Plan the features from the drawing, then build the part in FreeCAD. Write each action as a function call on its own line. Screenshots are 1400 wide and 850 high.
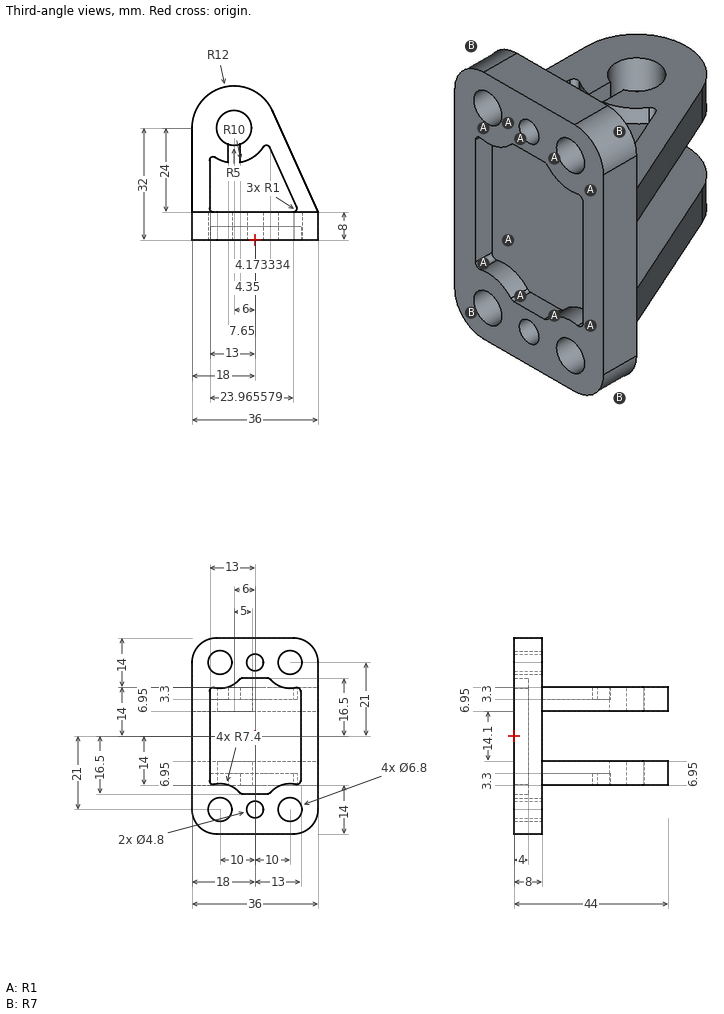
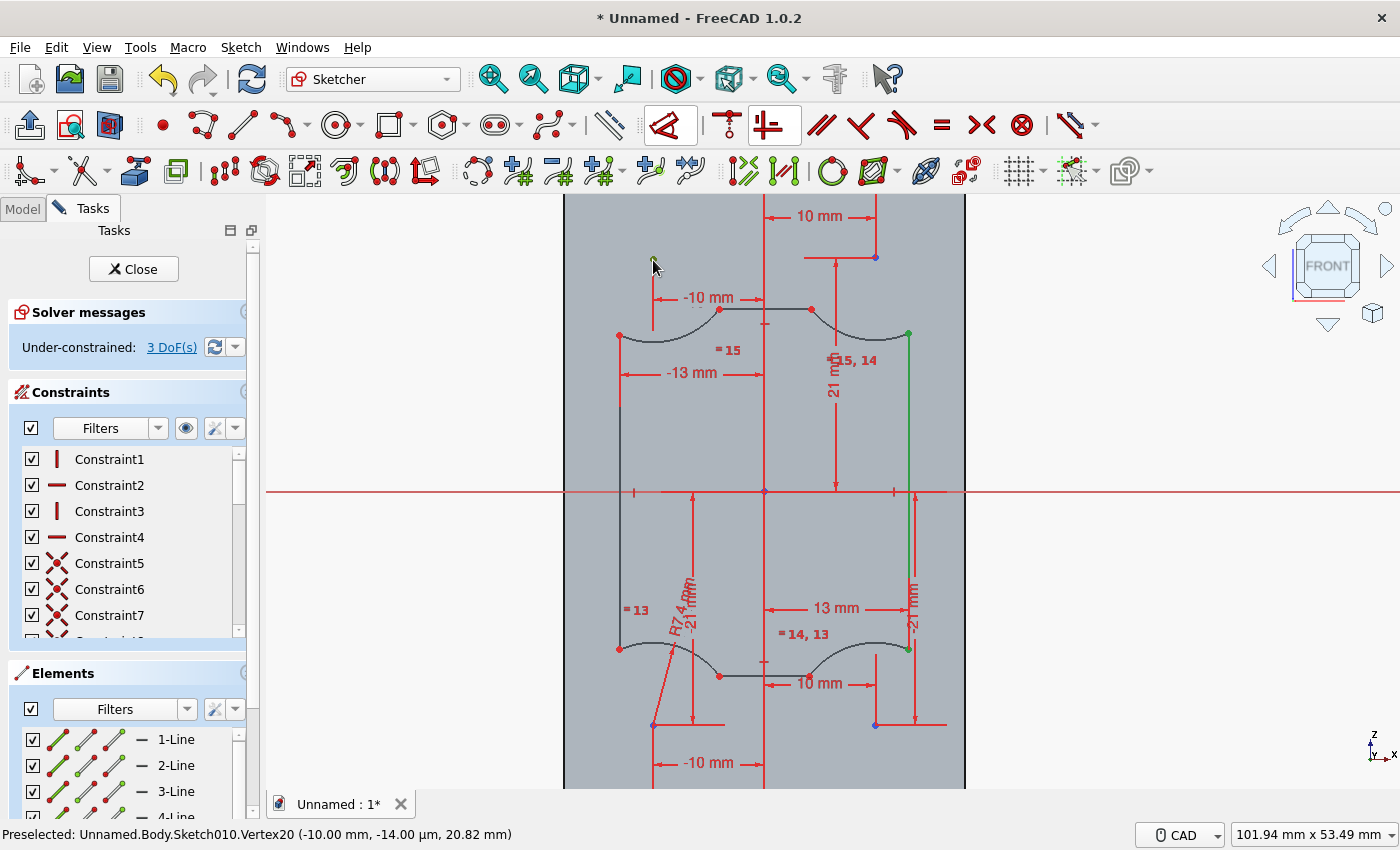
key(i)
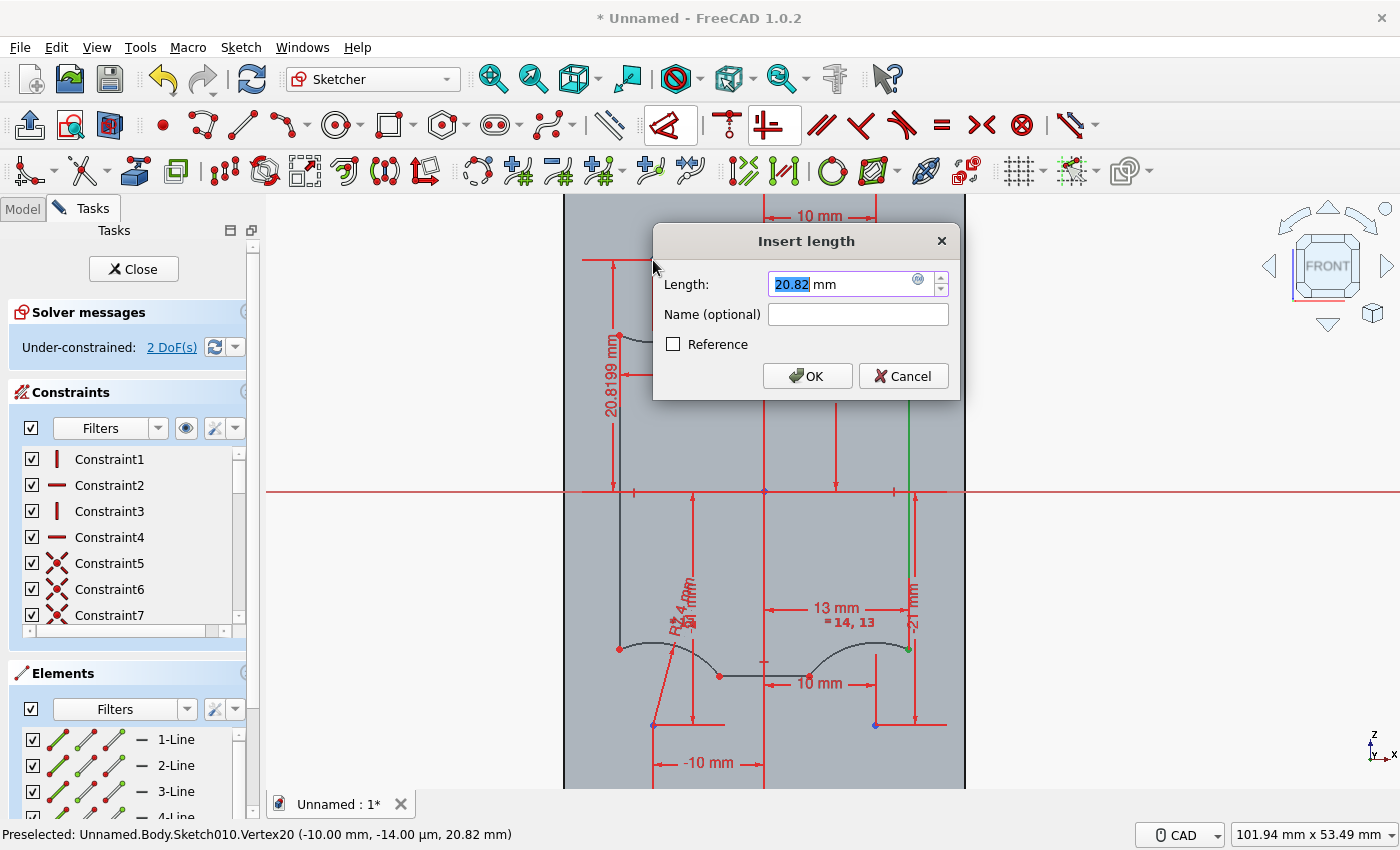
text(21)
key(Return)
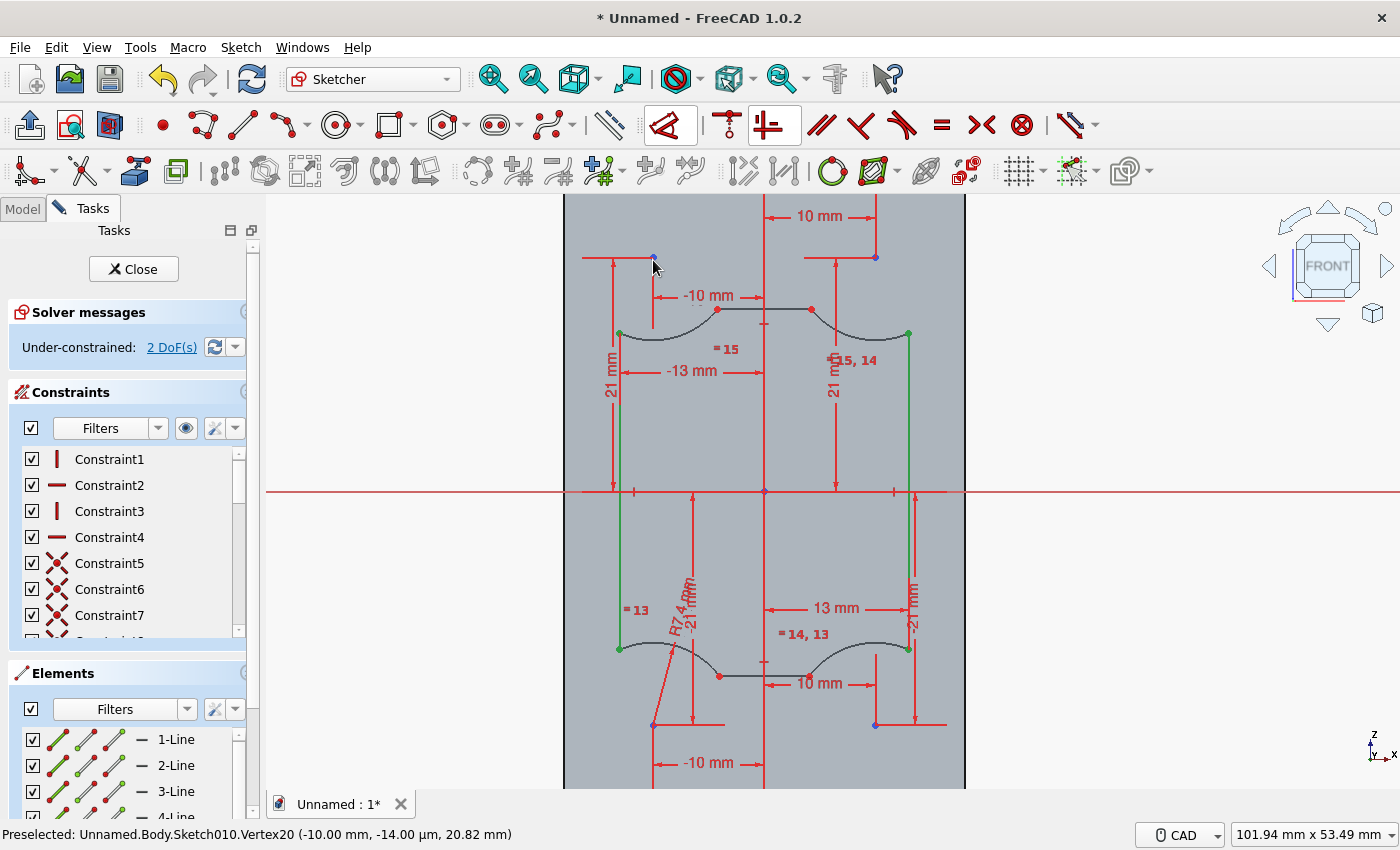
click(719, 676)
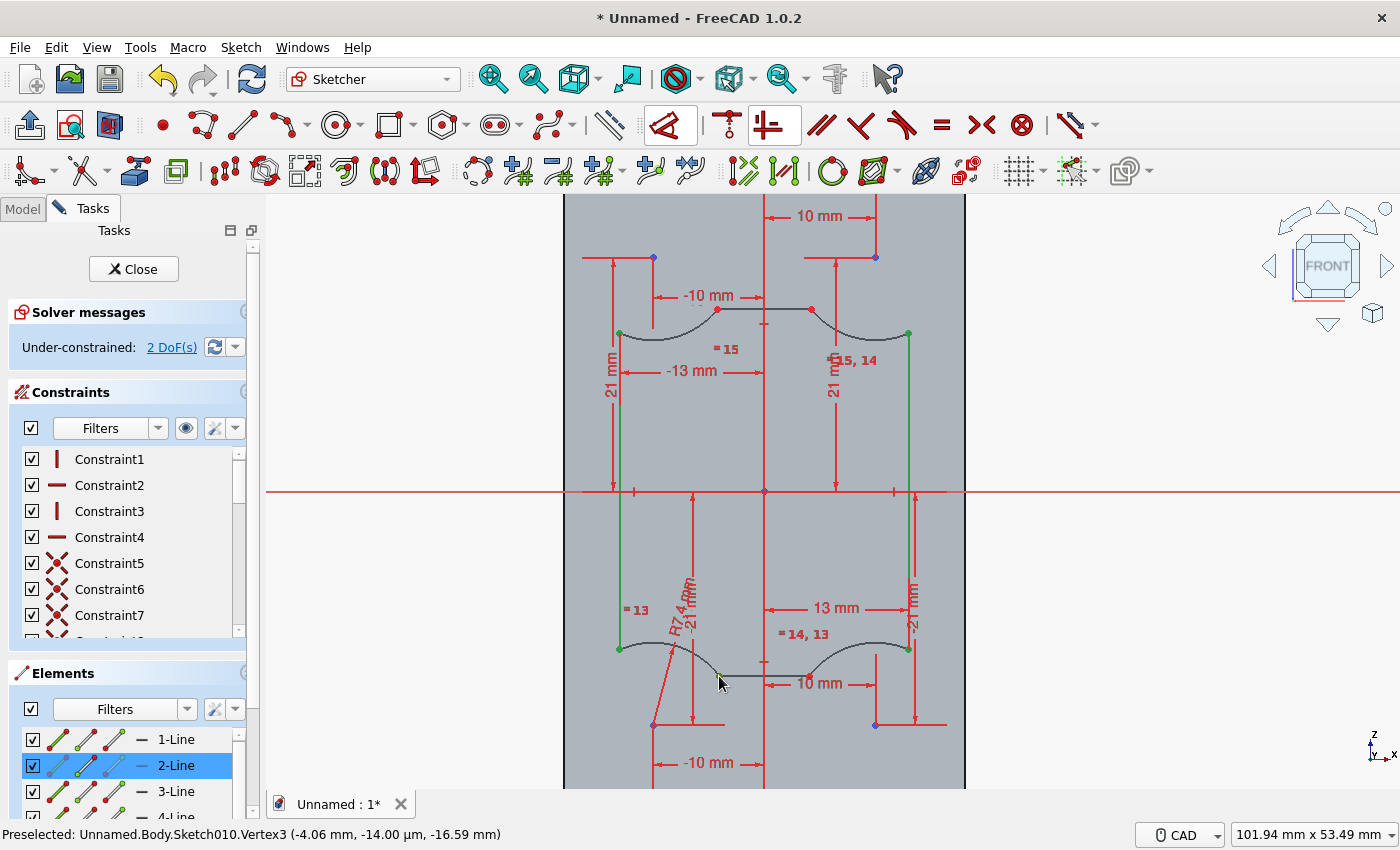
key(i)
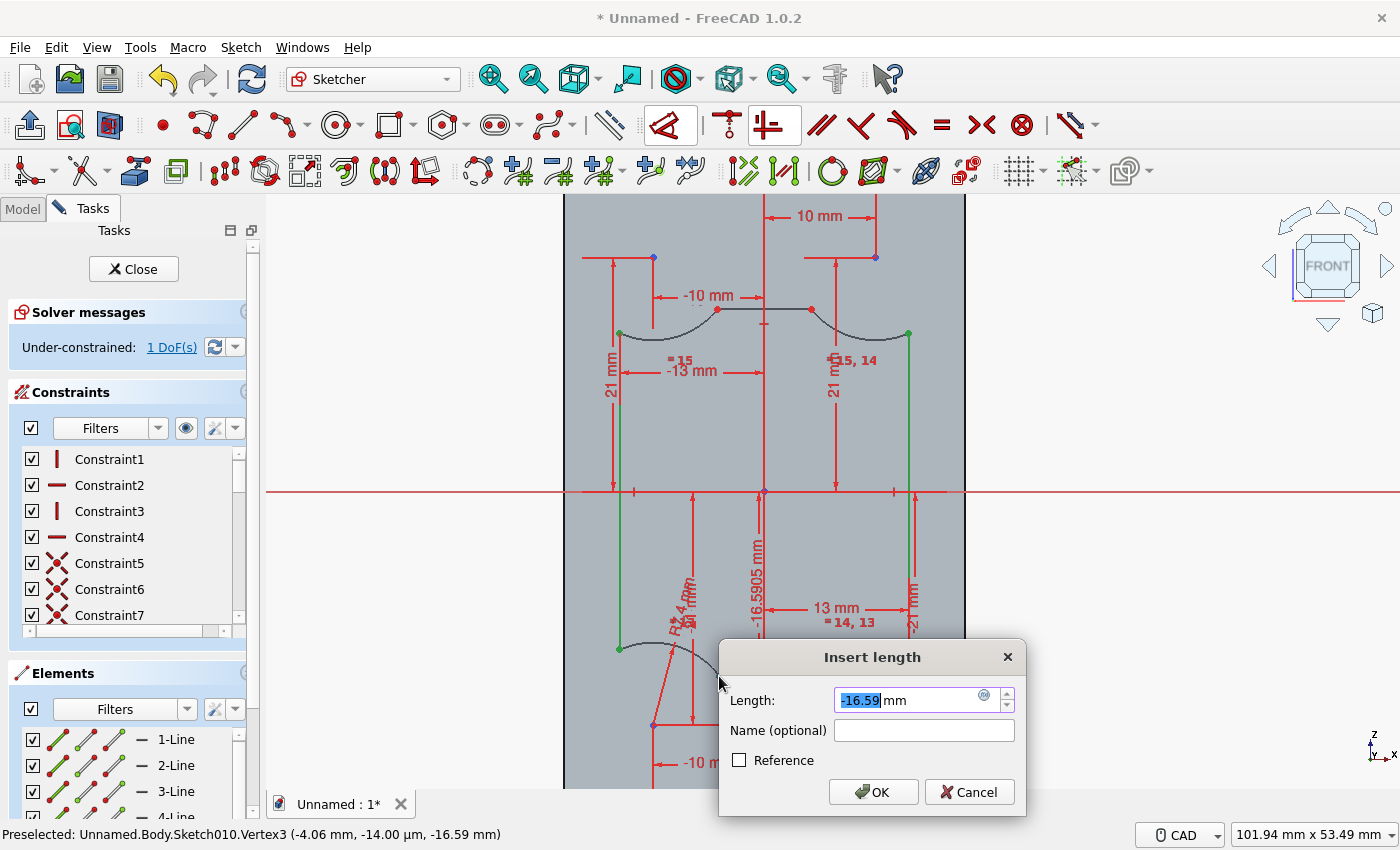
text(-16.5)
key(Return)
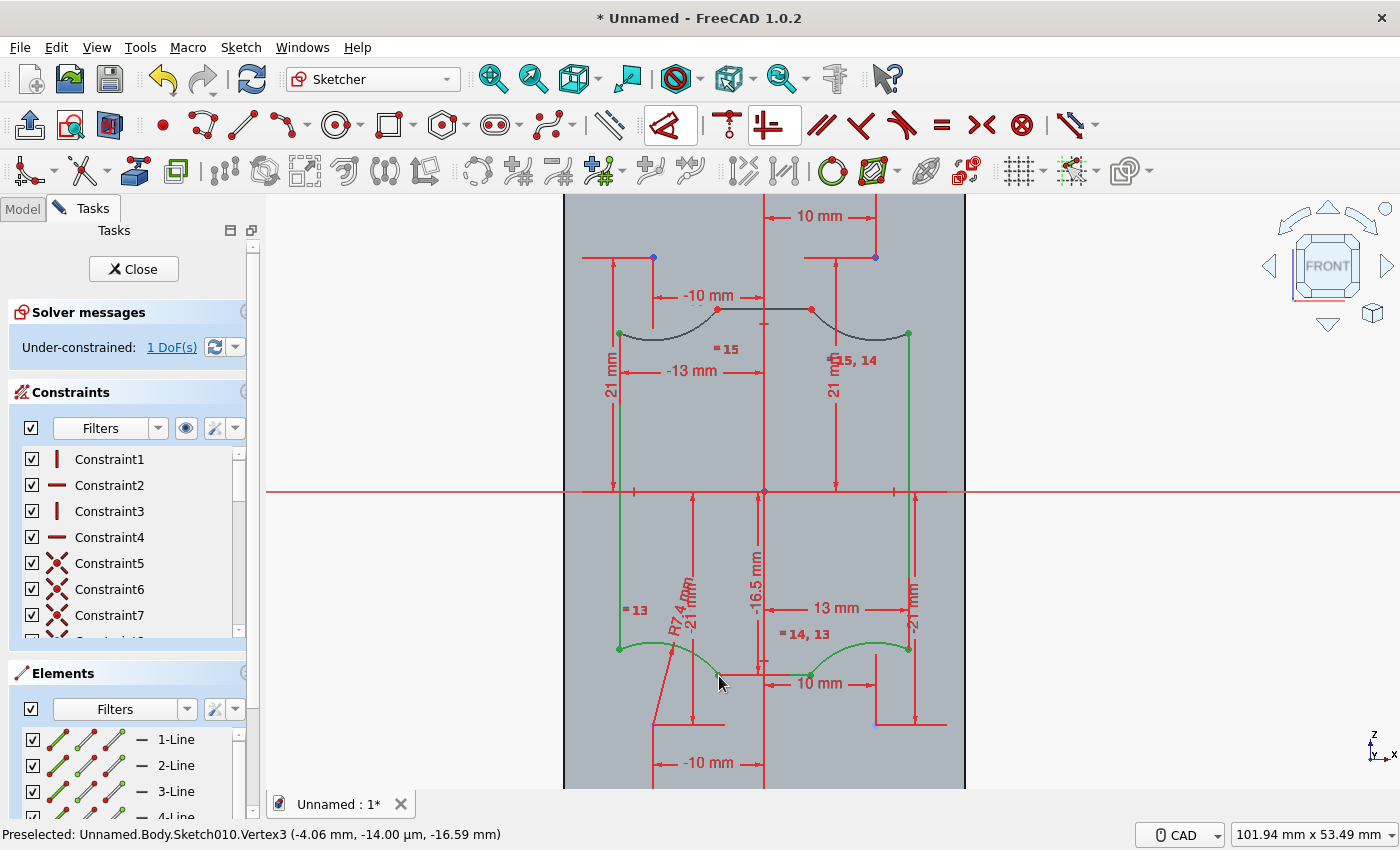
click(811, 309)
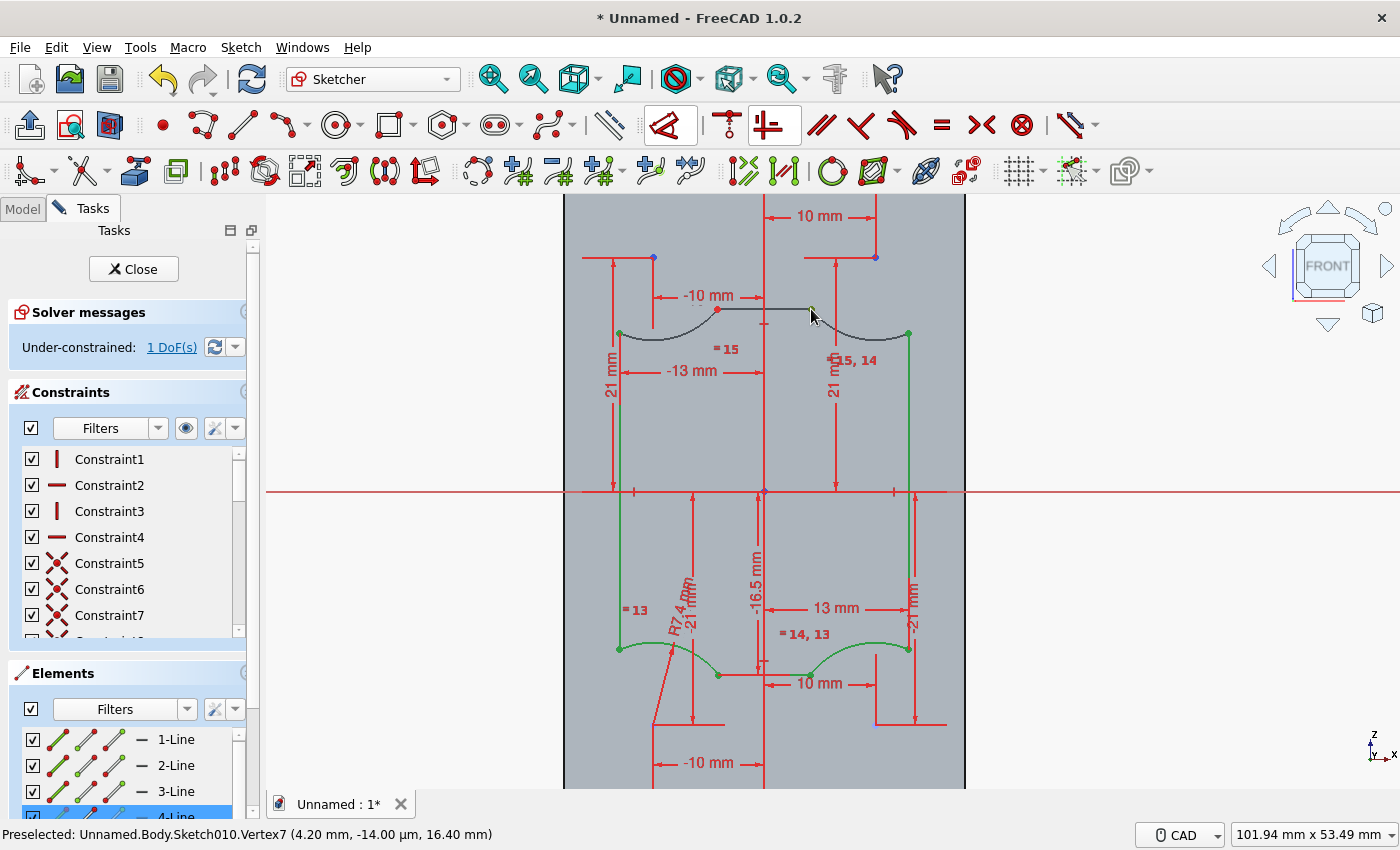
key(i)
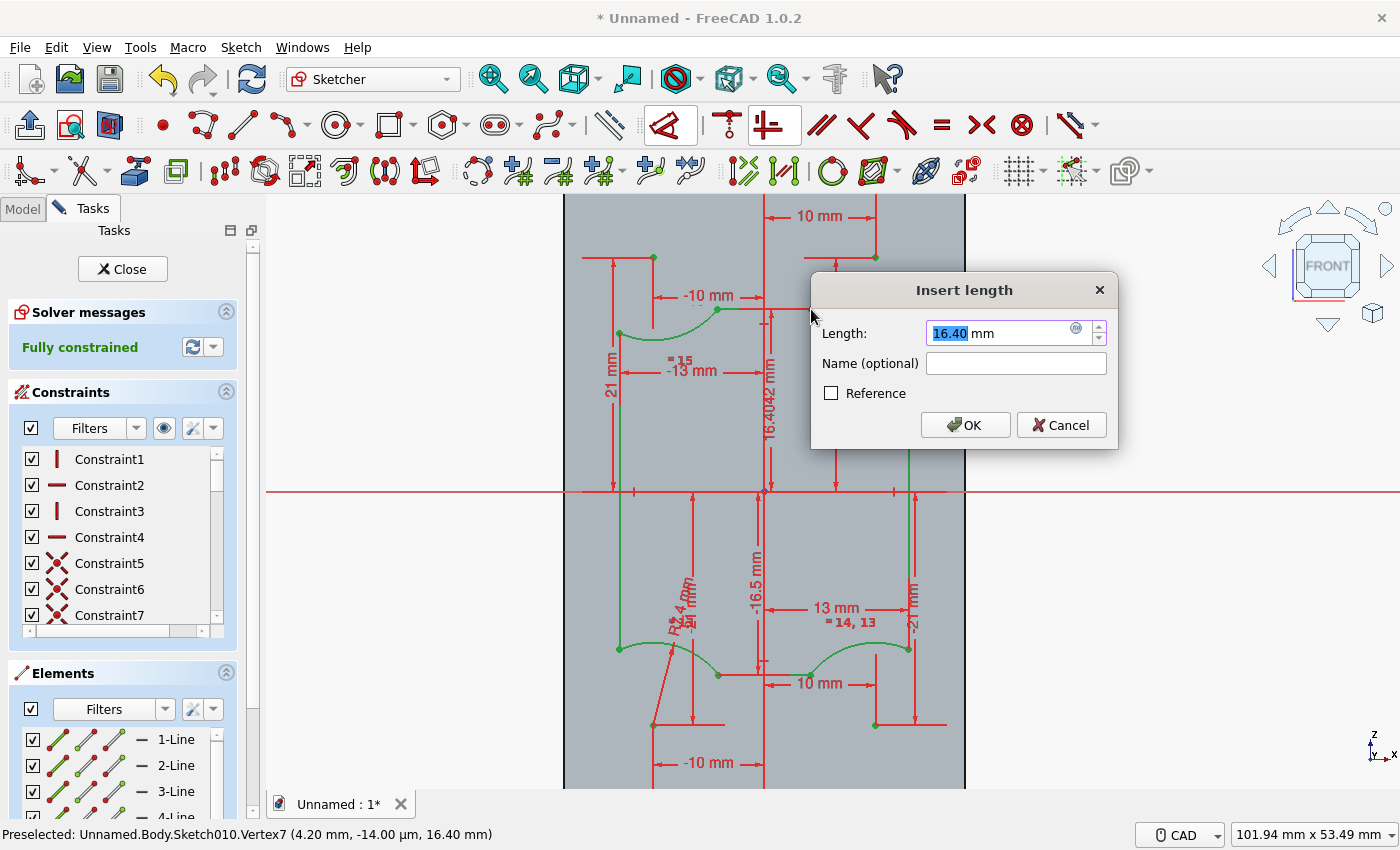
text(16.5)
key(Return)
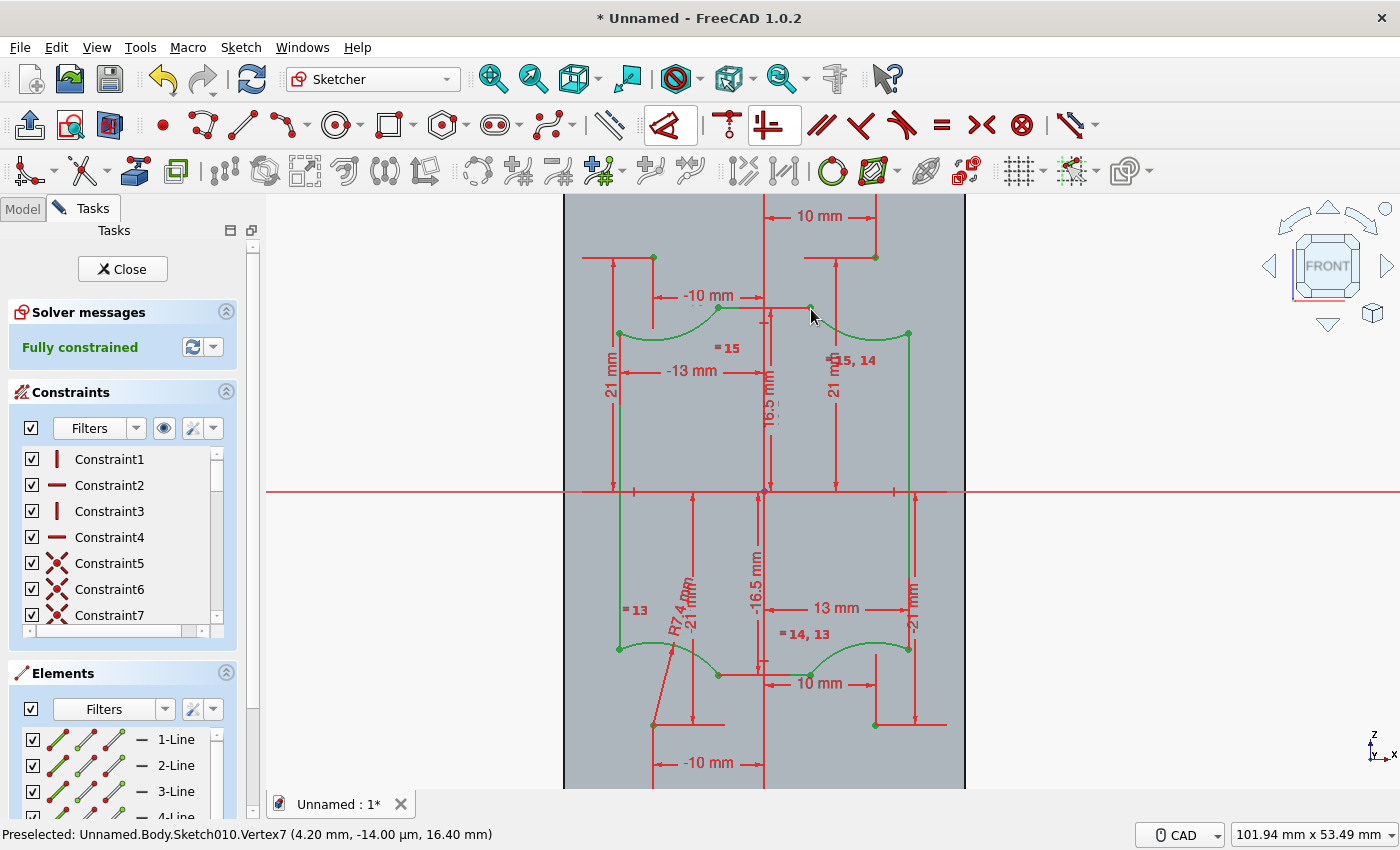
click(123, 269)